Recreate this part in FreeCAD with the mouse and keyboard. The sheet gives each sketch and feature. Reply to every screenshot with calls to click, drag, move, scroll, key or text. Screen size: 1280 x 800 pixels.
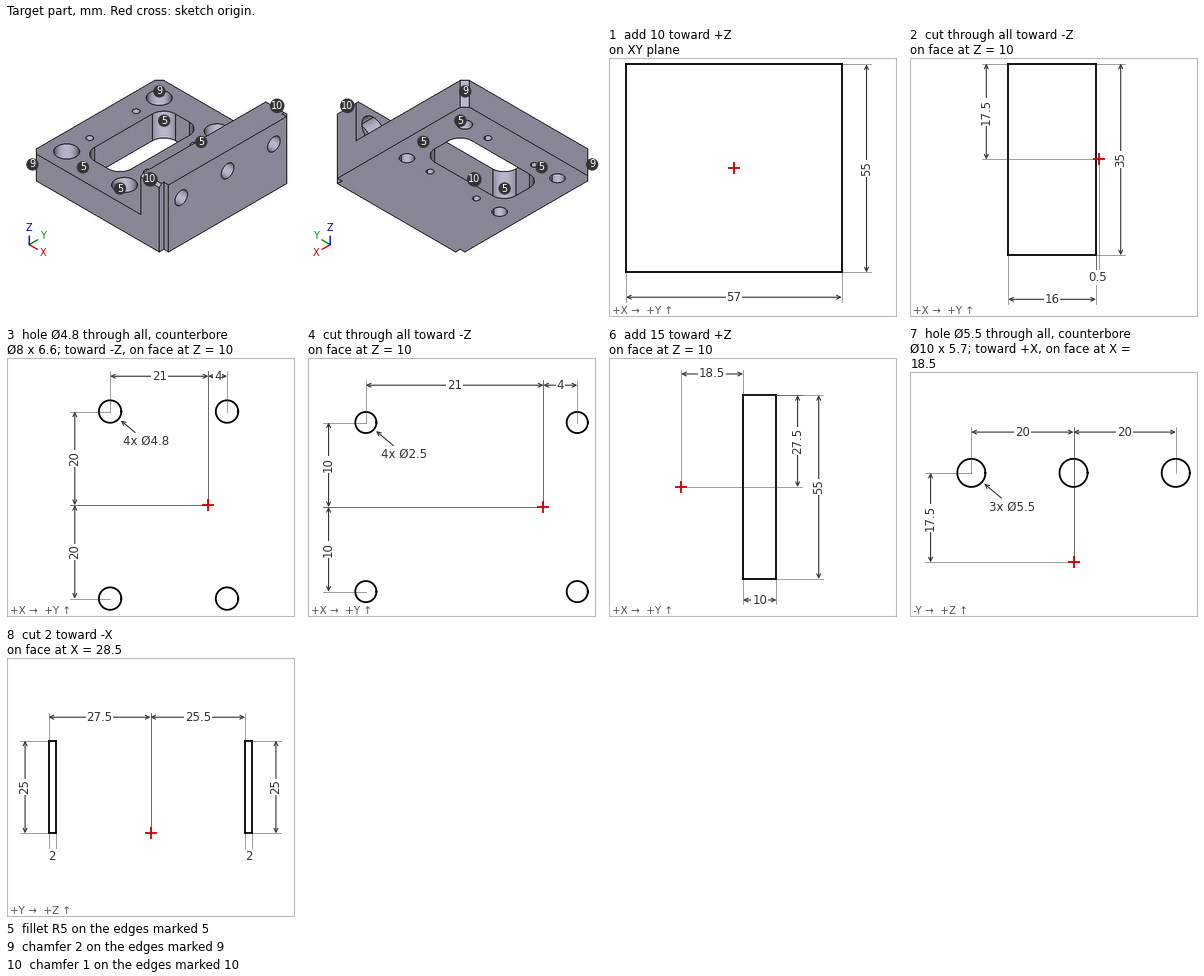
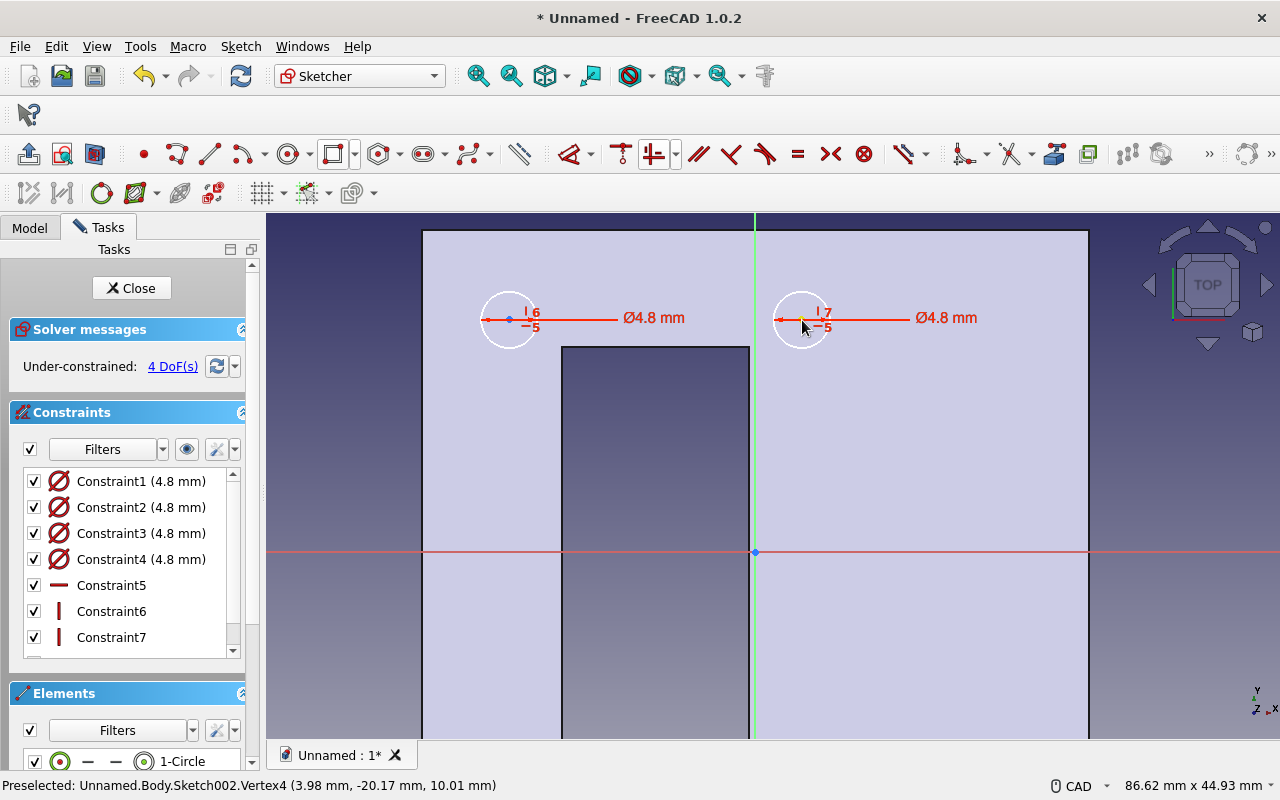
click(802, 320)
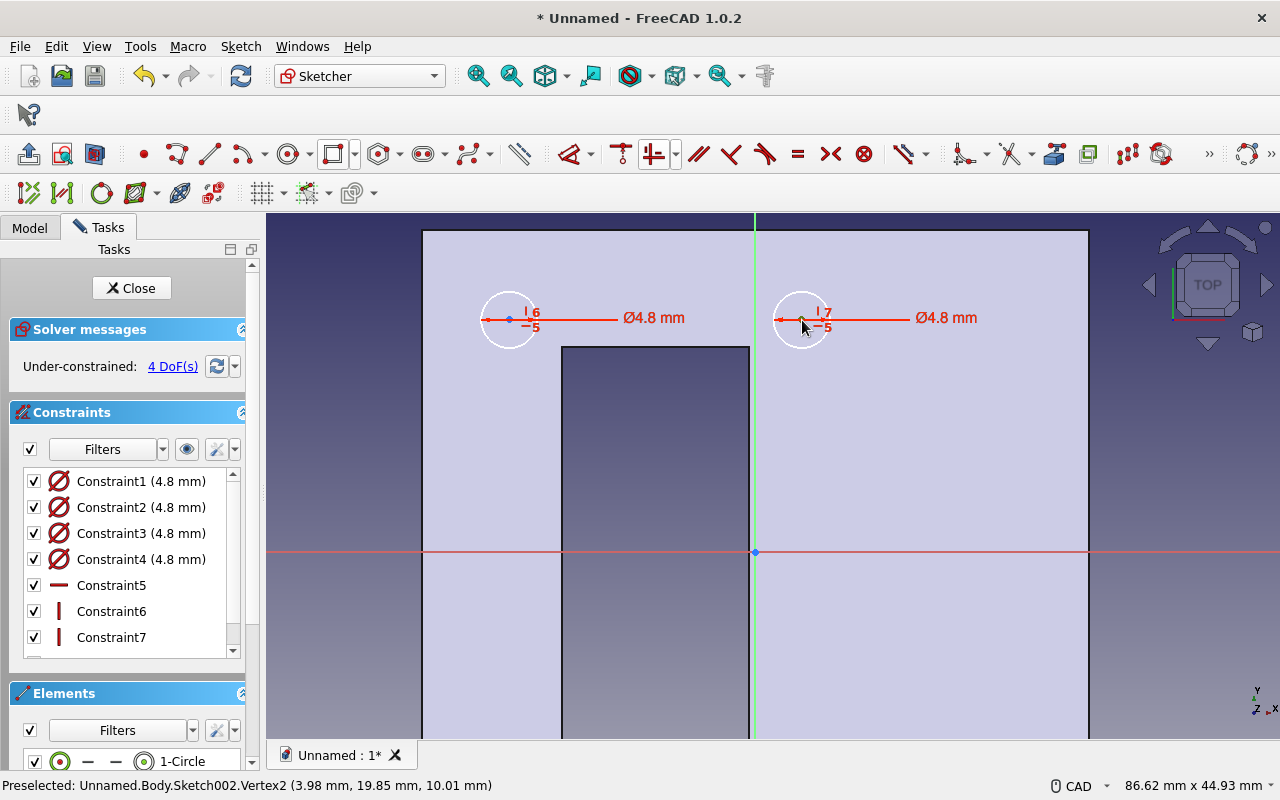
click(590, 154)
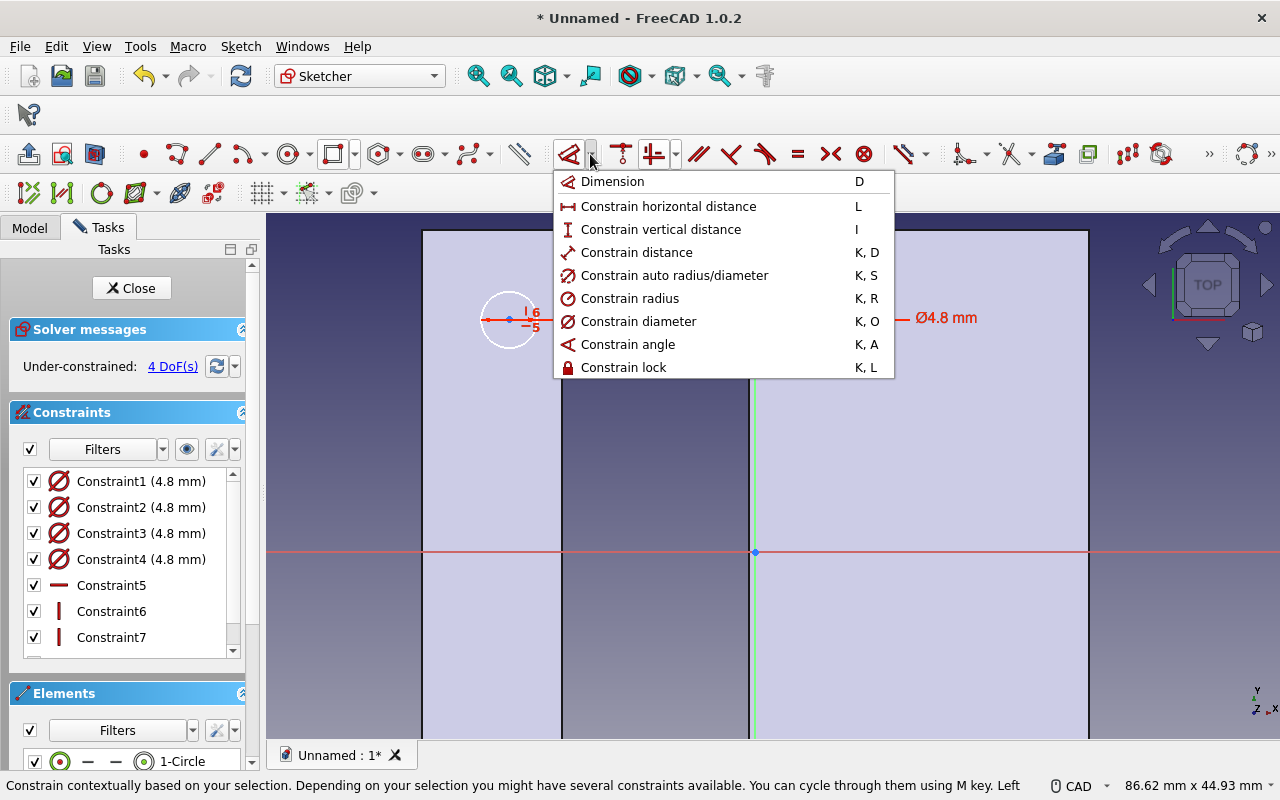
click(724, 206)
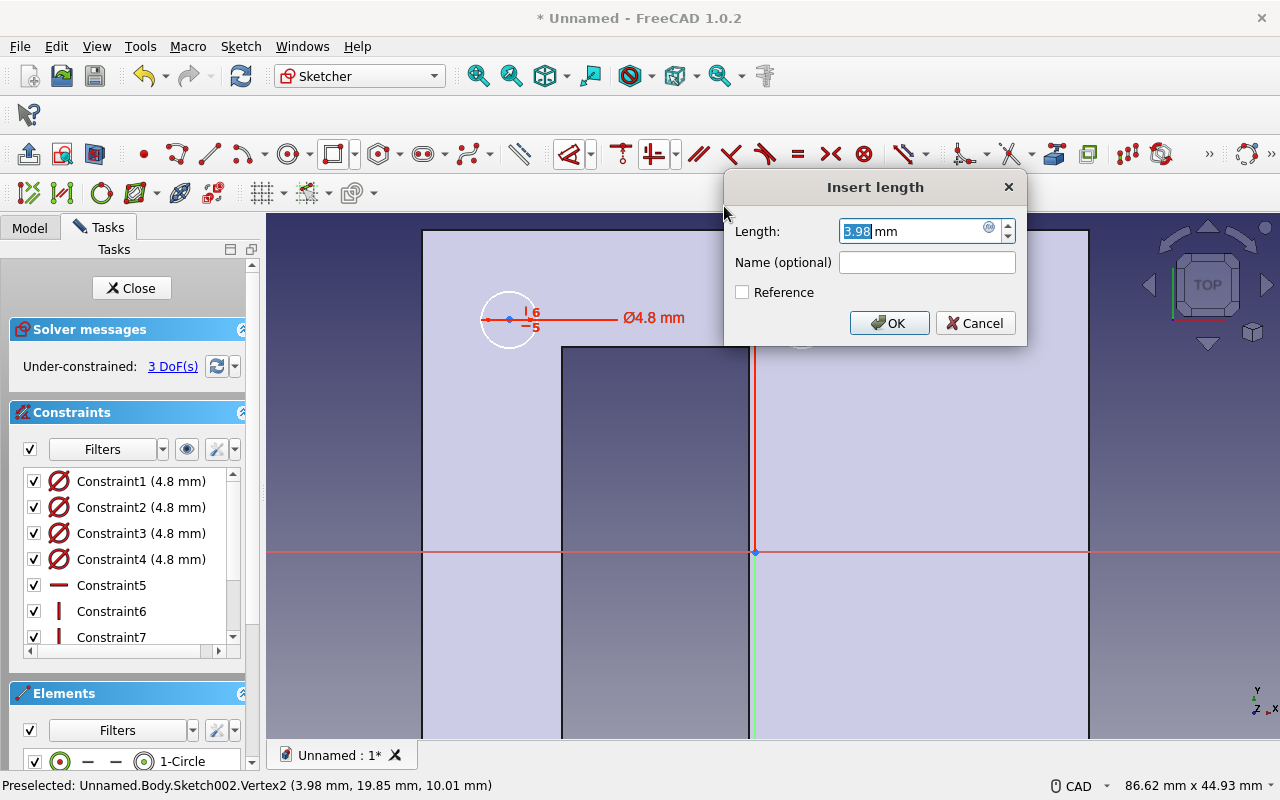
text(4)
key(Return)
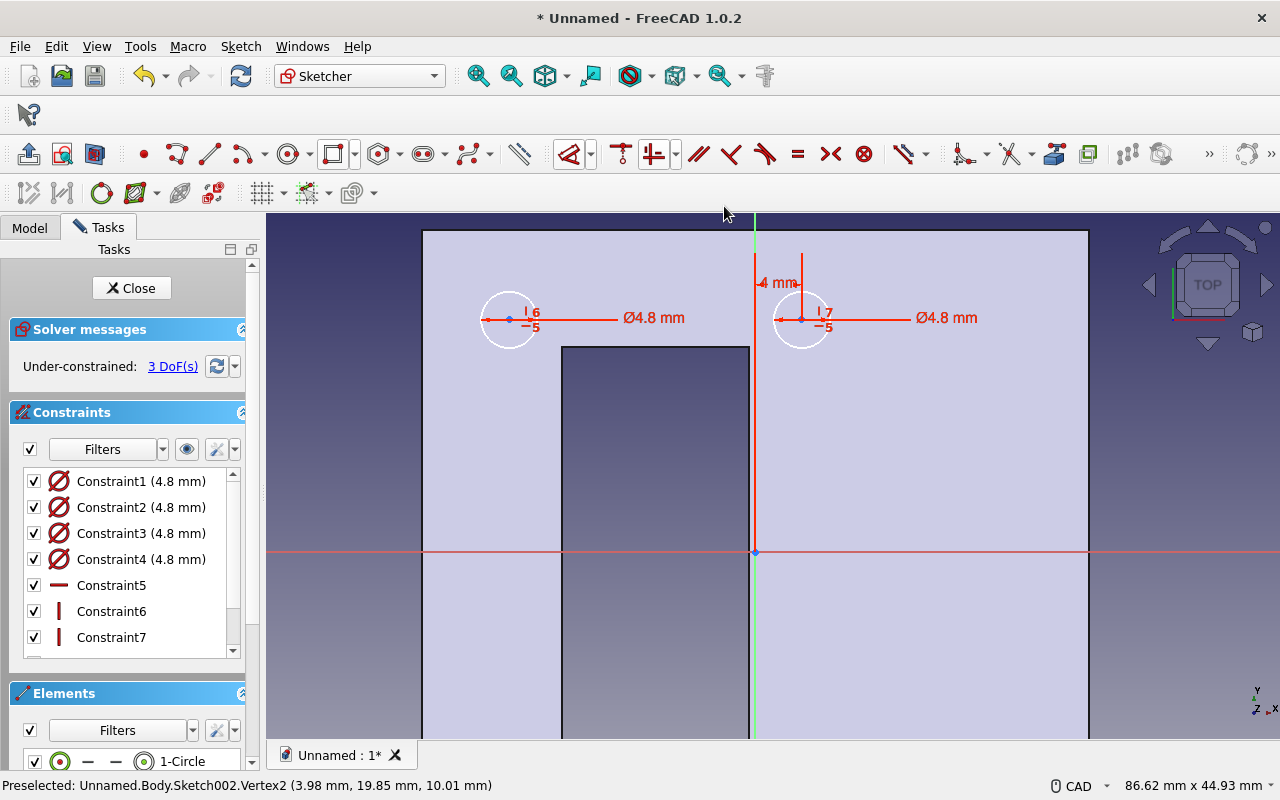
click(509, 320)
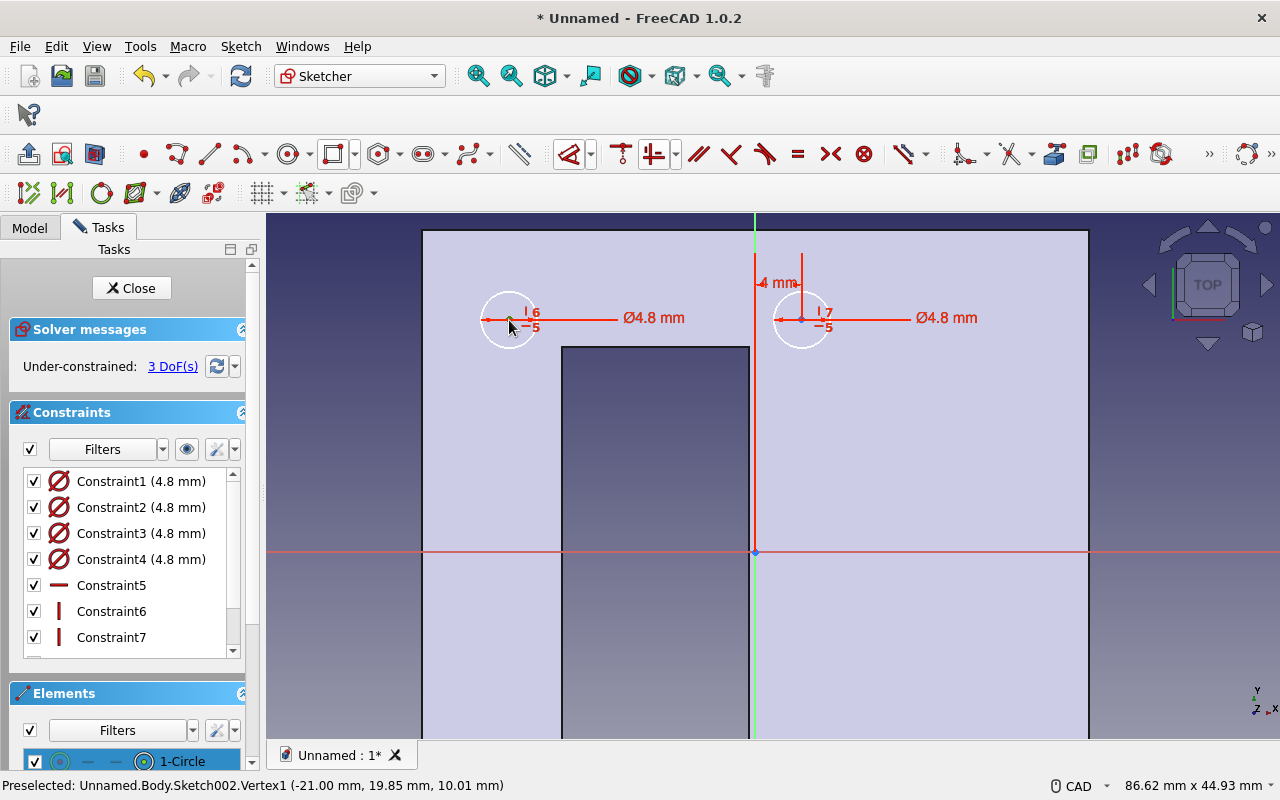
click(590, 154)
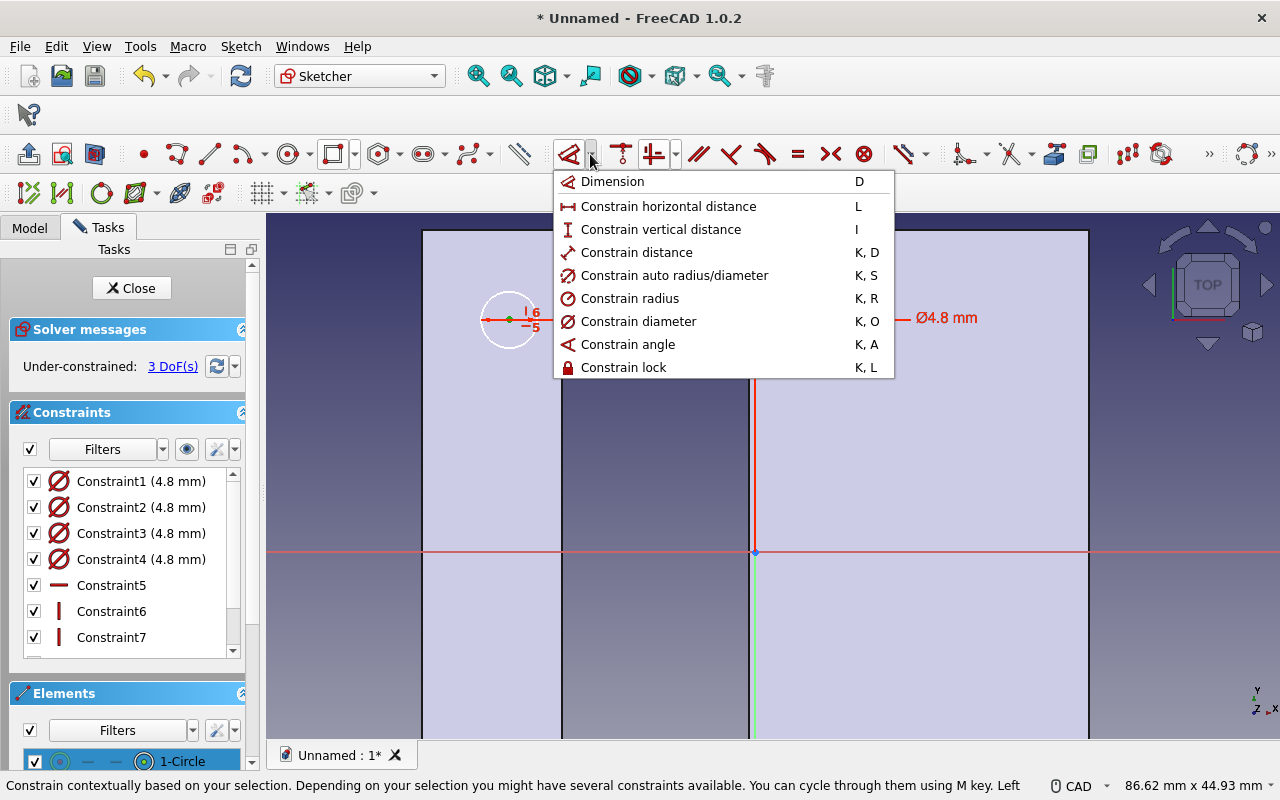
click(724, 206)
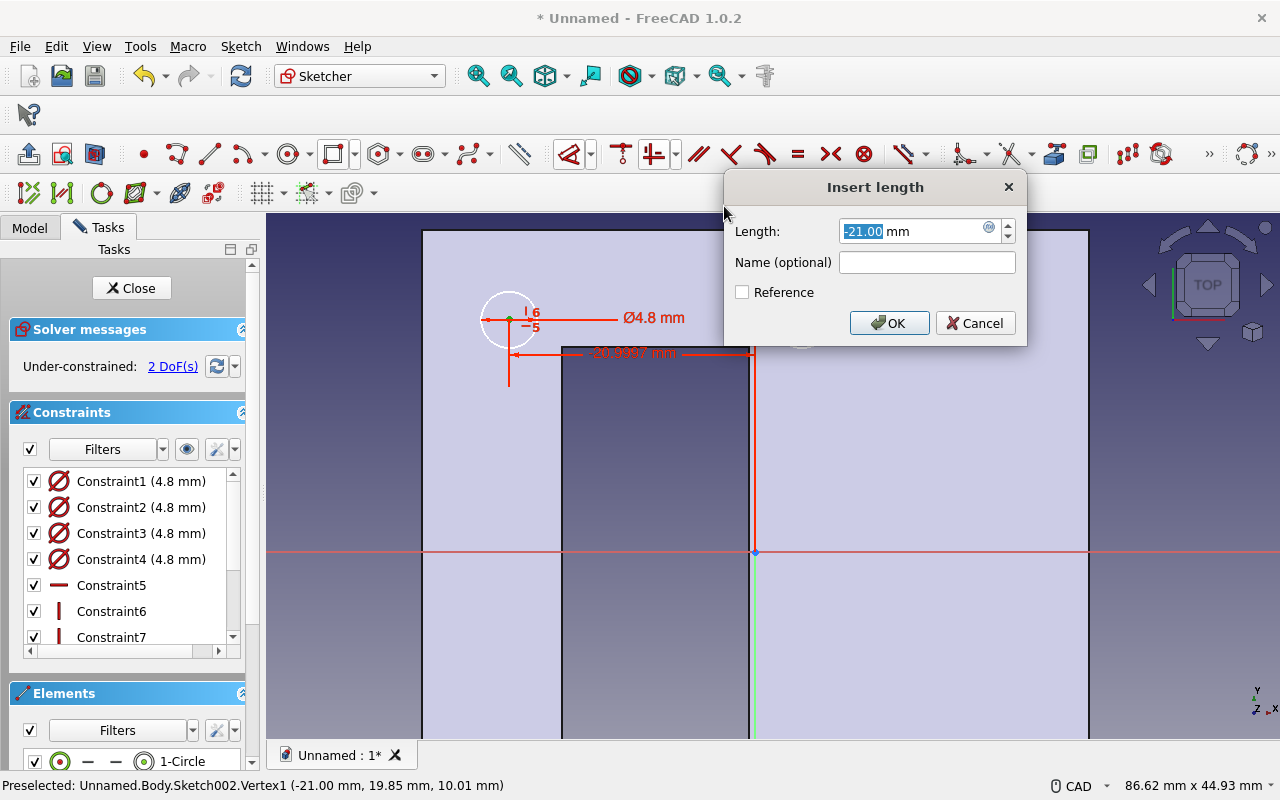
text(-21)
key(Return)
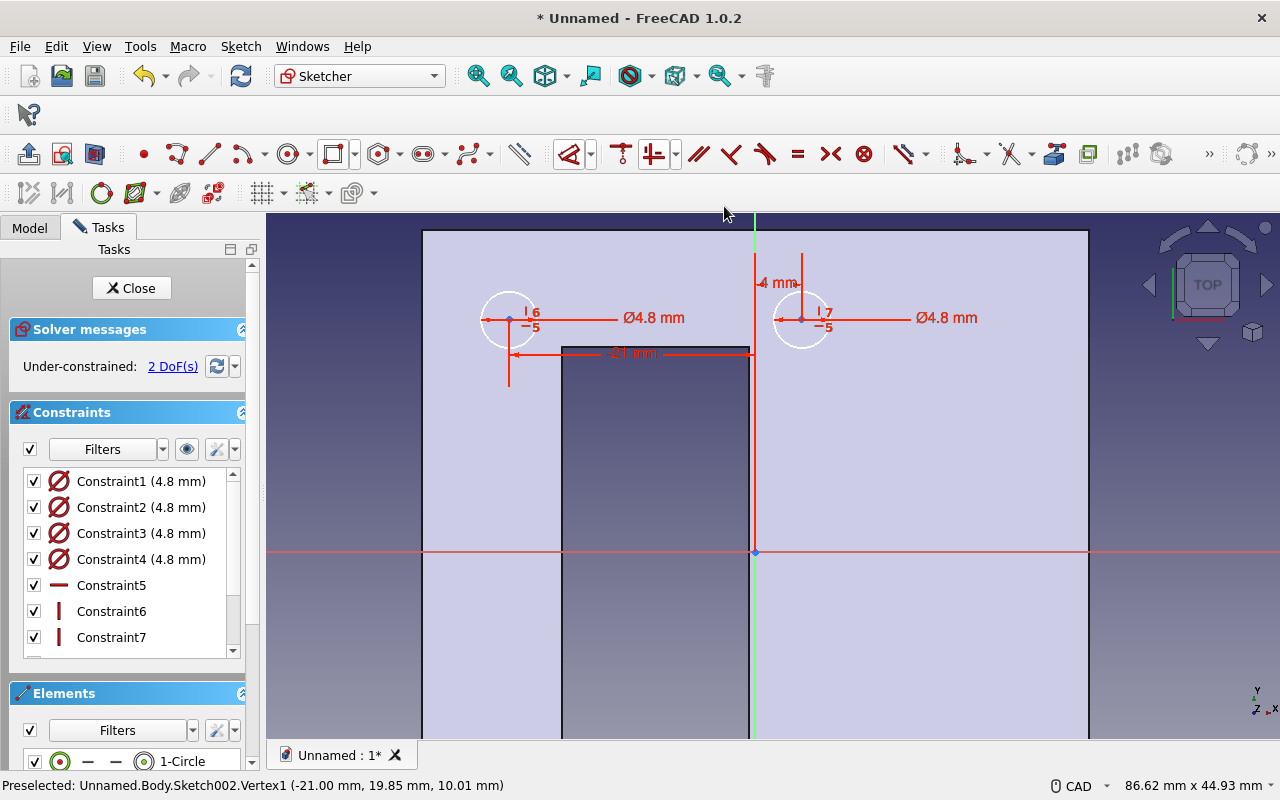
click(509, 320)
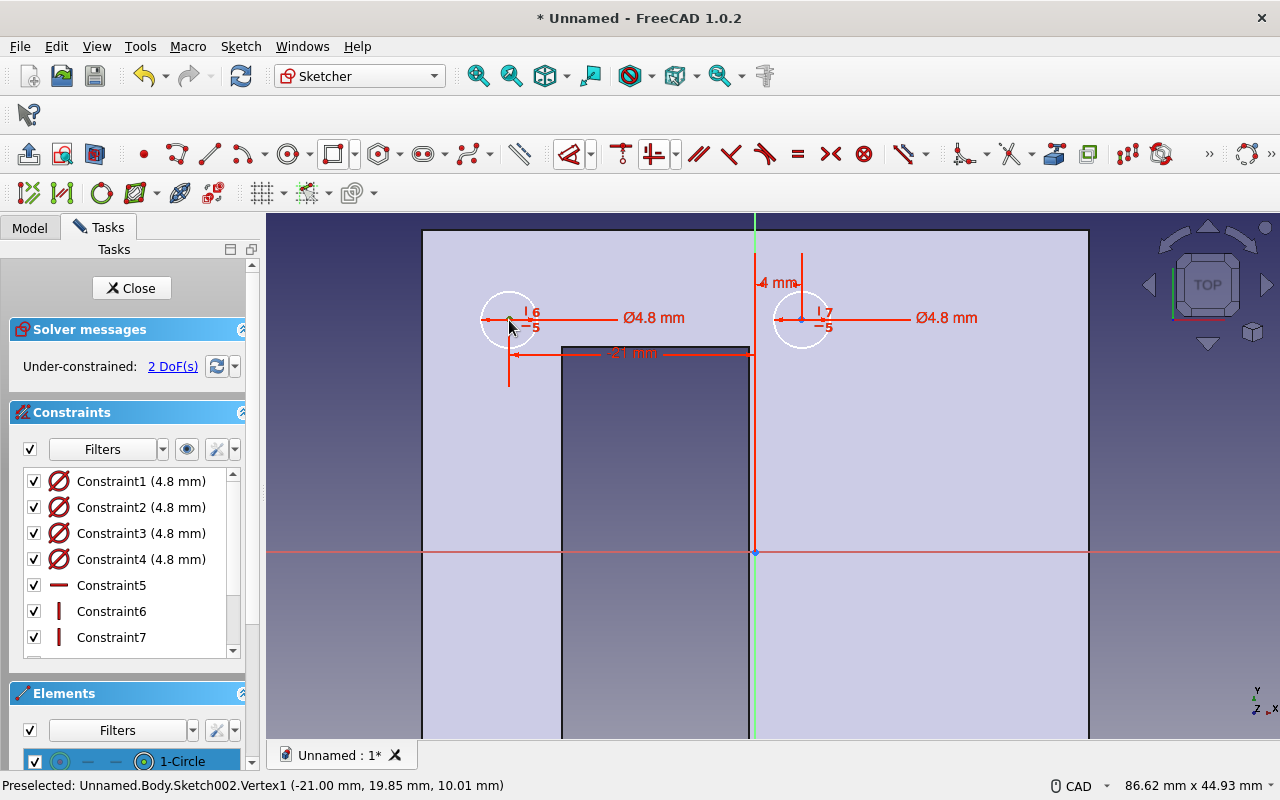
click(590, 154)